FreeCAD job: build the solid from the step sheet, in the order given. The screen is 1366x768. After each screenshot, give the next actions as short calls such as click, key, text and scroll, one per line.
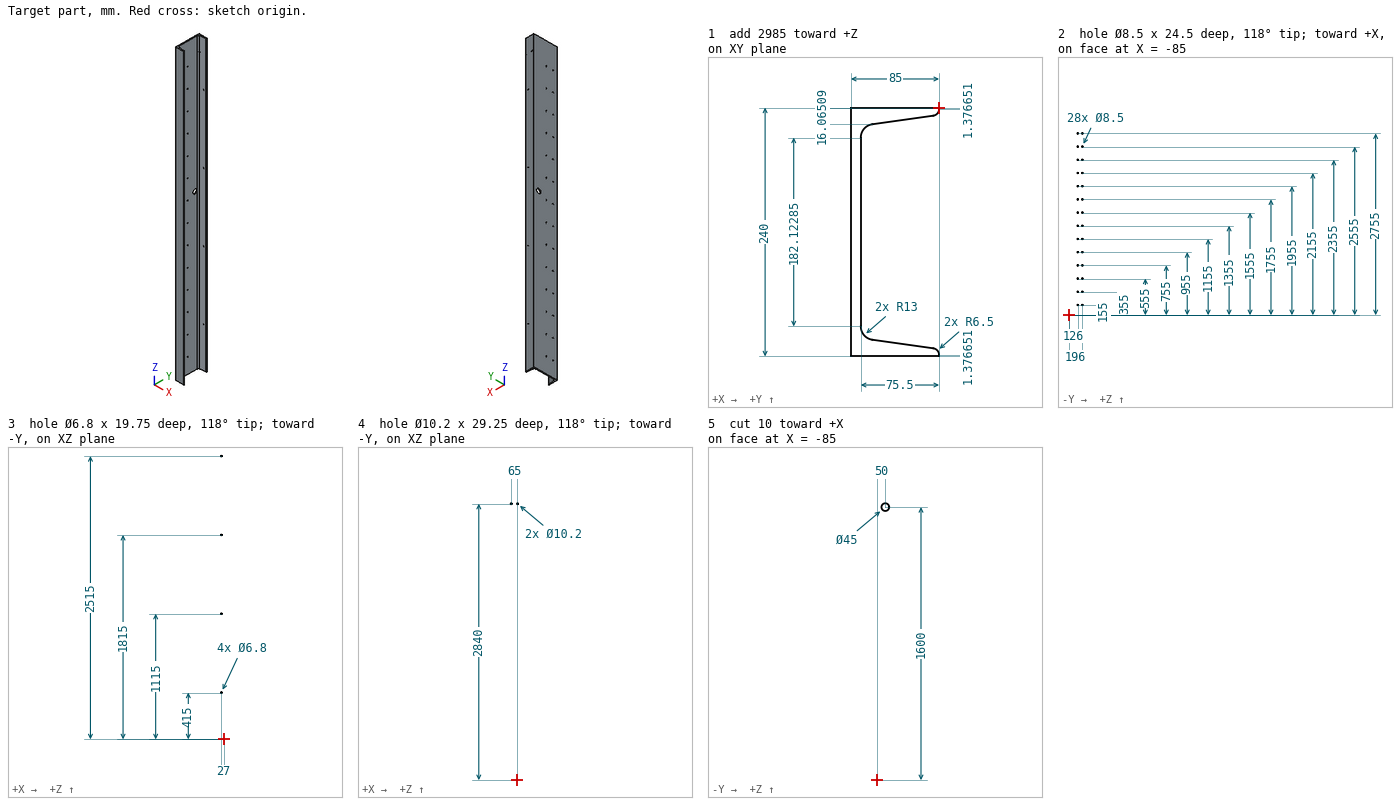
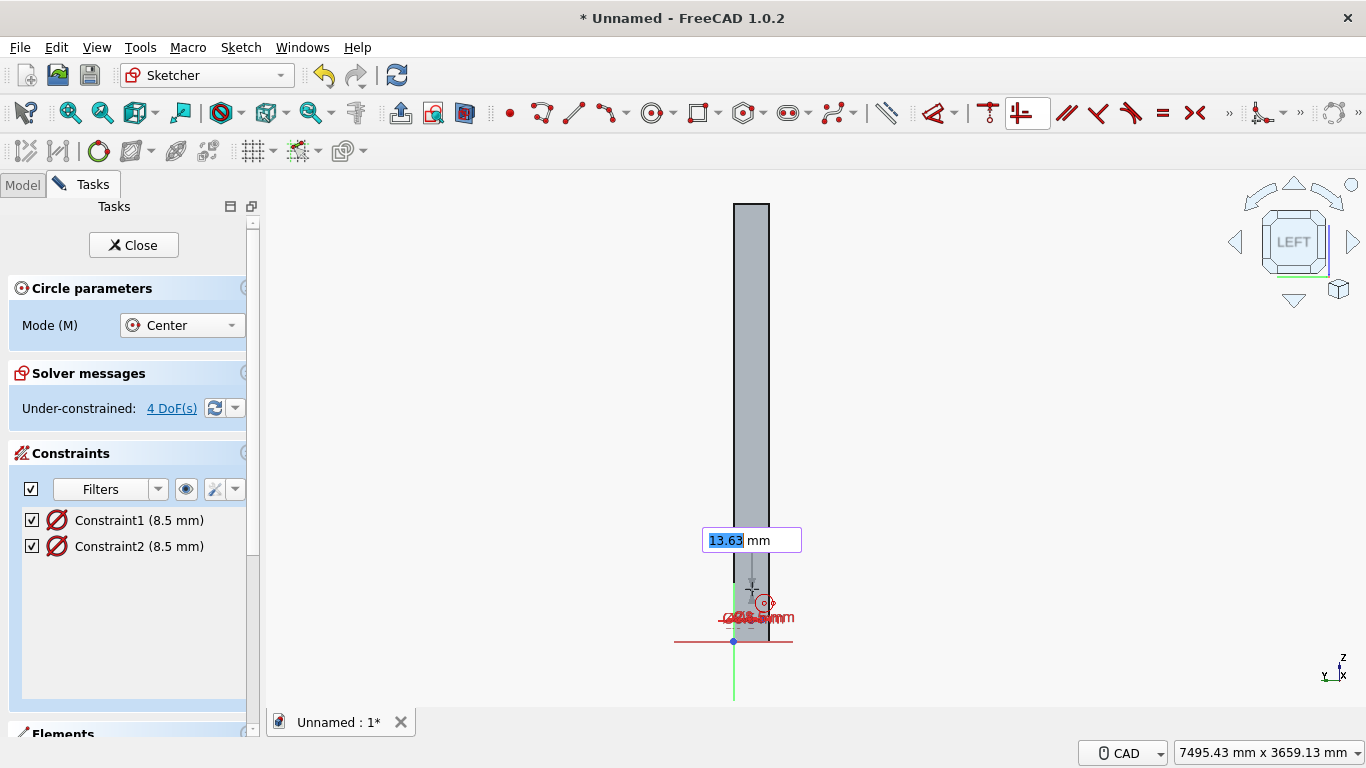
text(8.5)
key(Return)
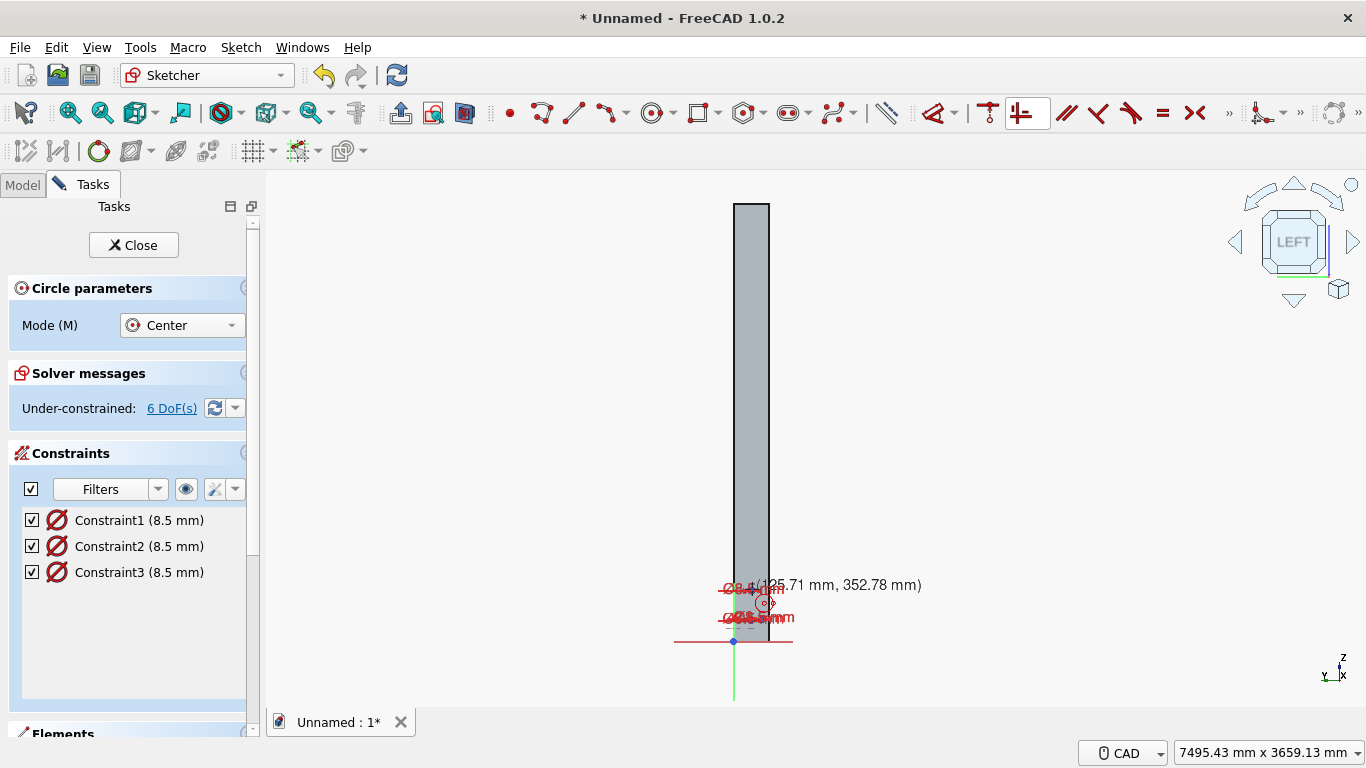
scroll(762, 590, up, 18)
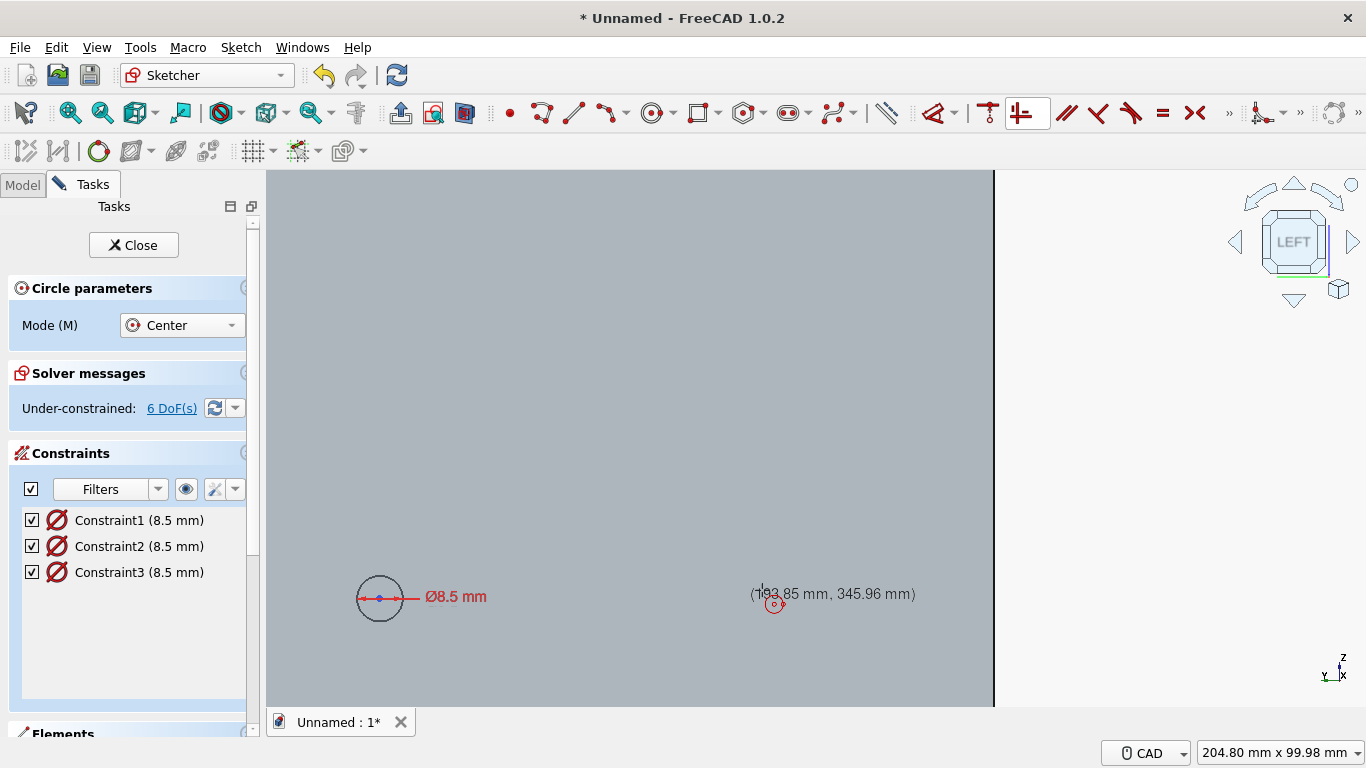
scroll(762, 590, down, 18)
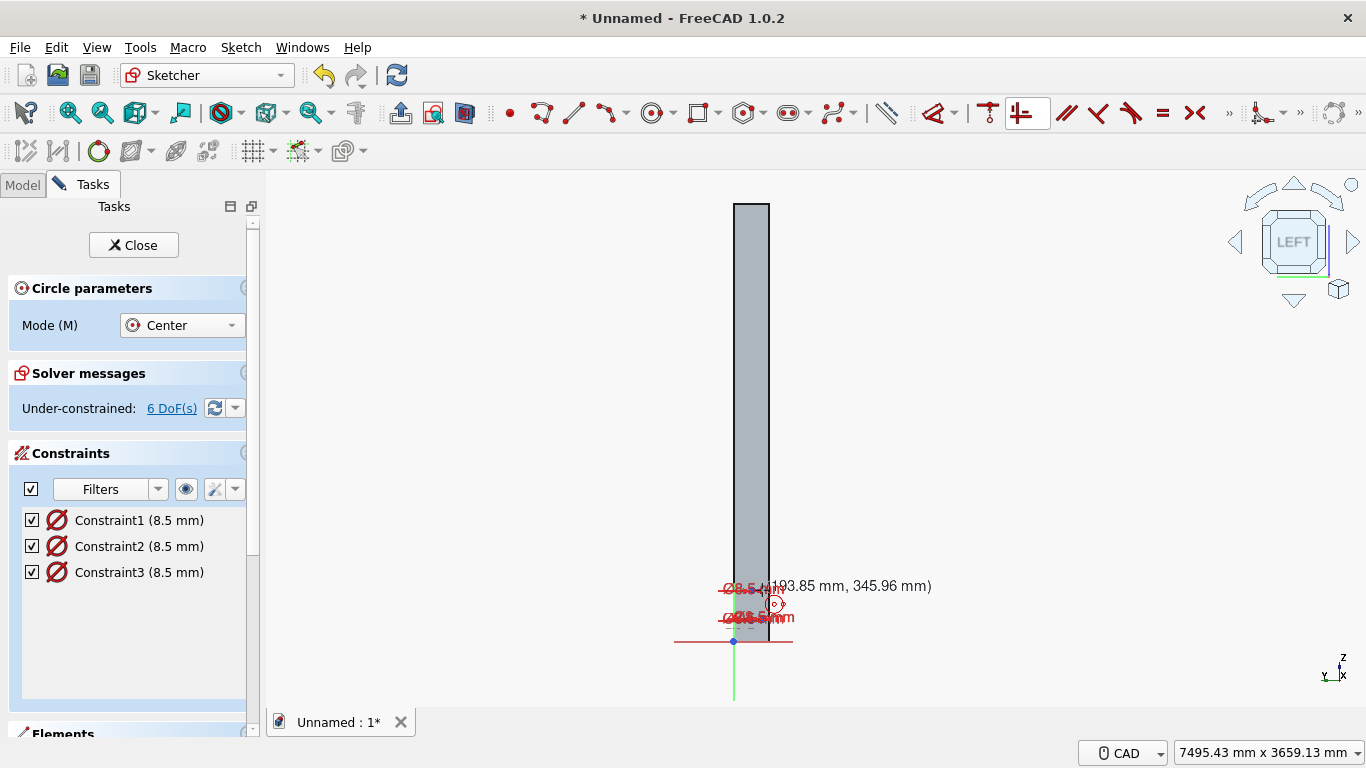
scroll(762, 590, up, 3)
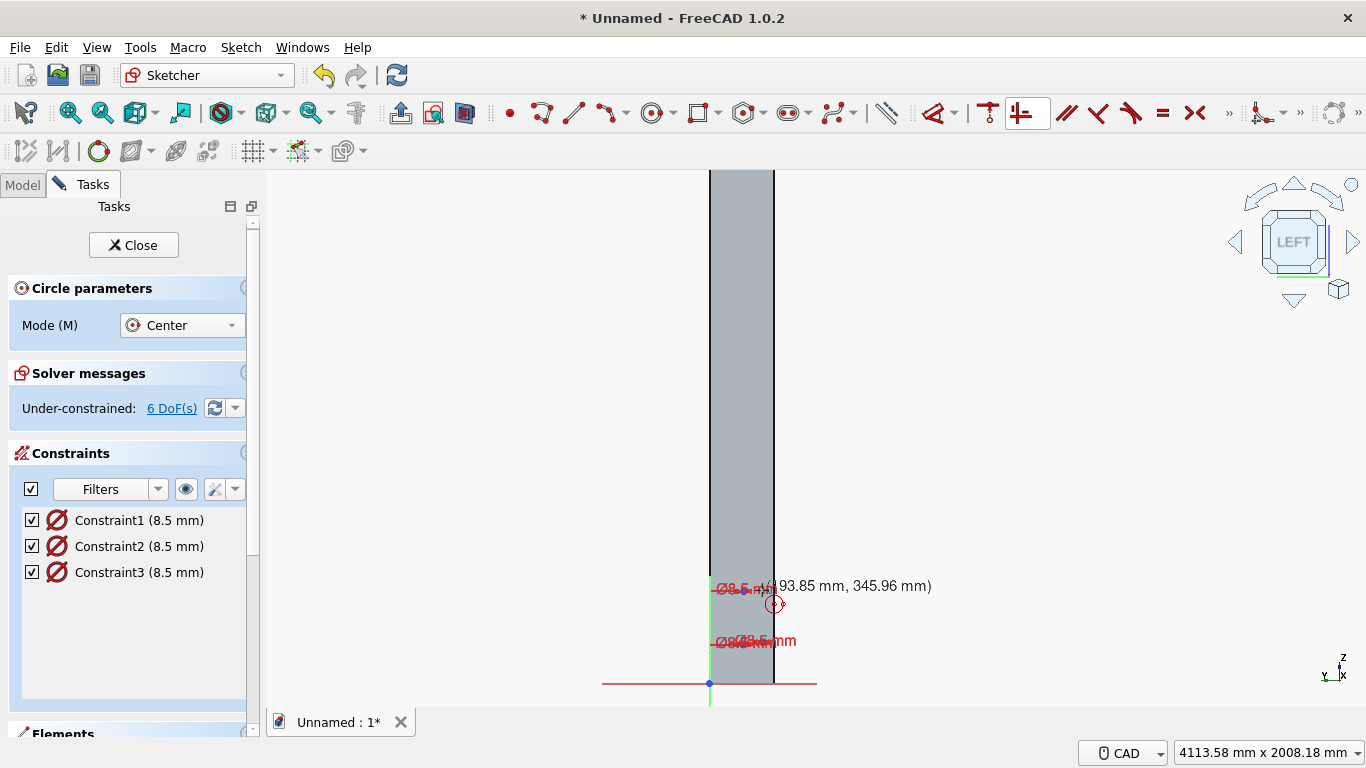
click(762, 589)
move(763, 588)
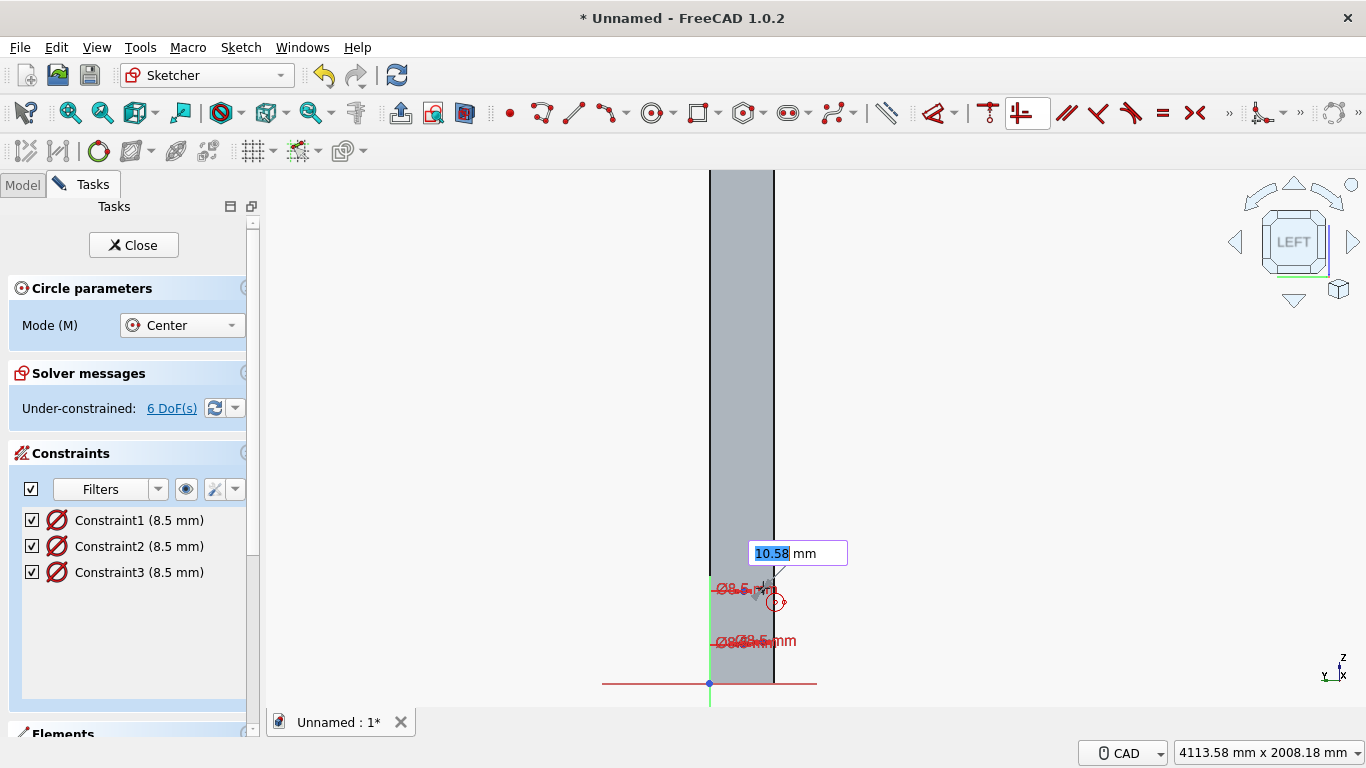
text(8.5)
key(Return)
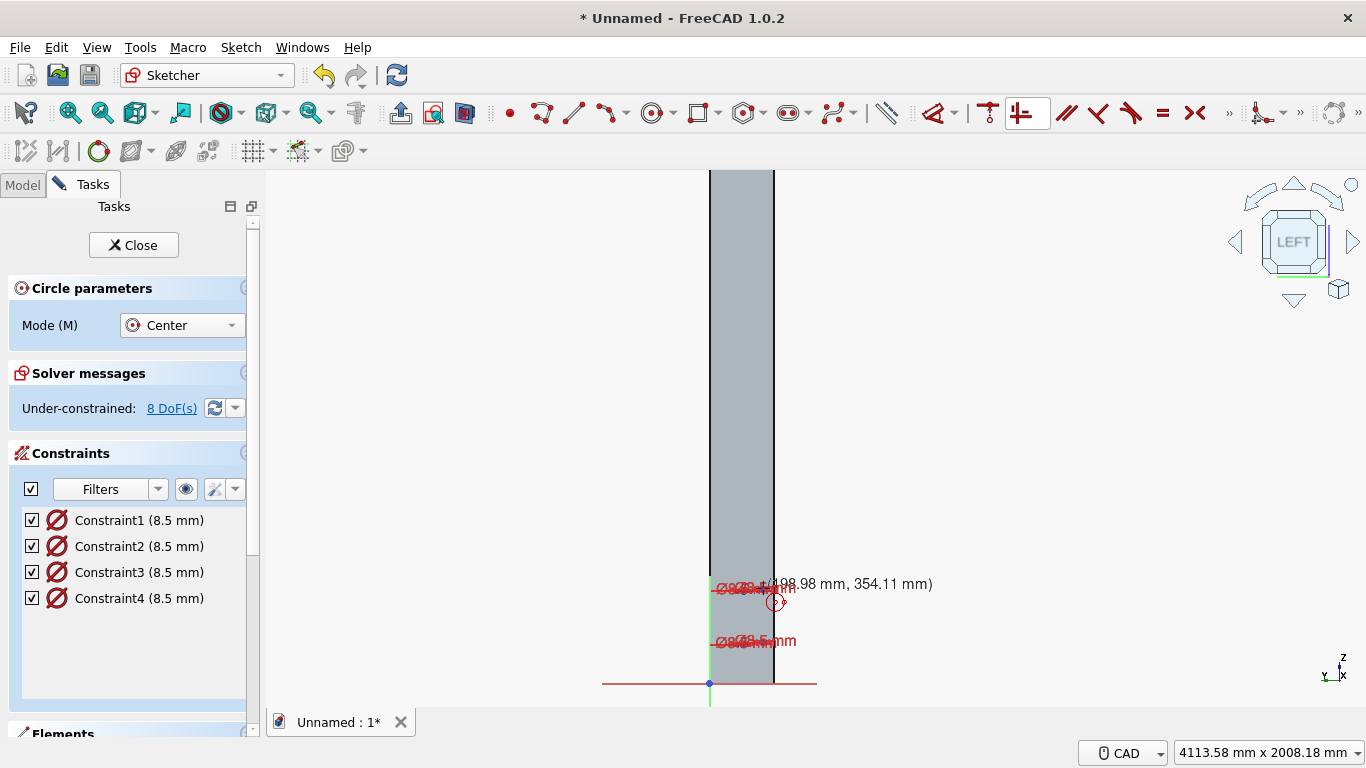
scroll(743, 535, up, 15)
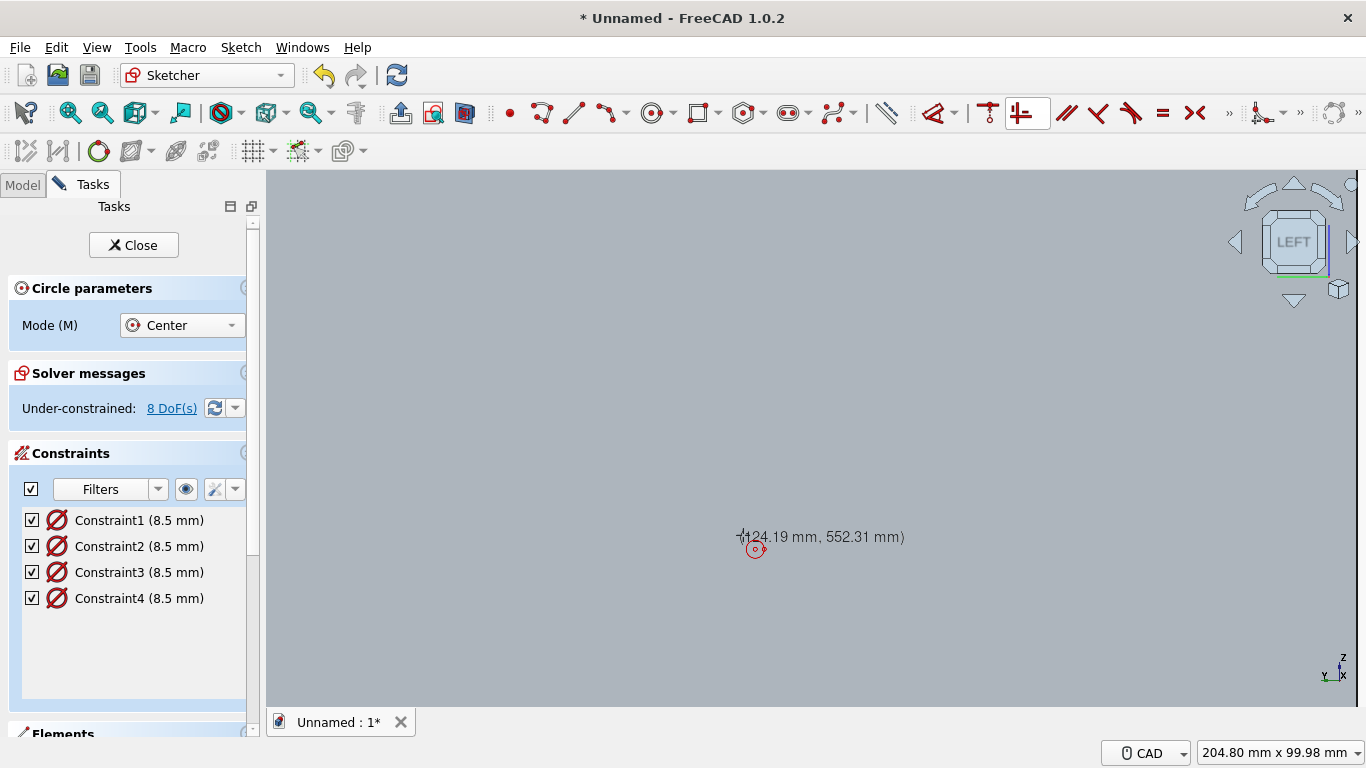
scroll(751, 560, down, 18)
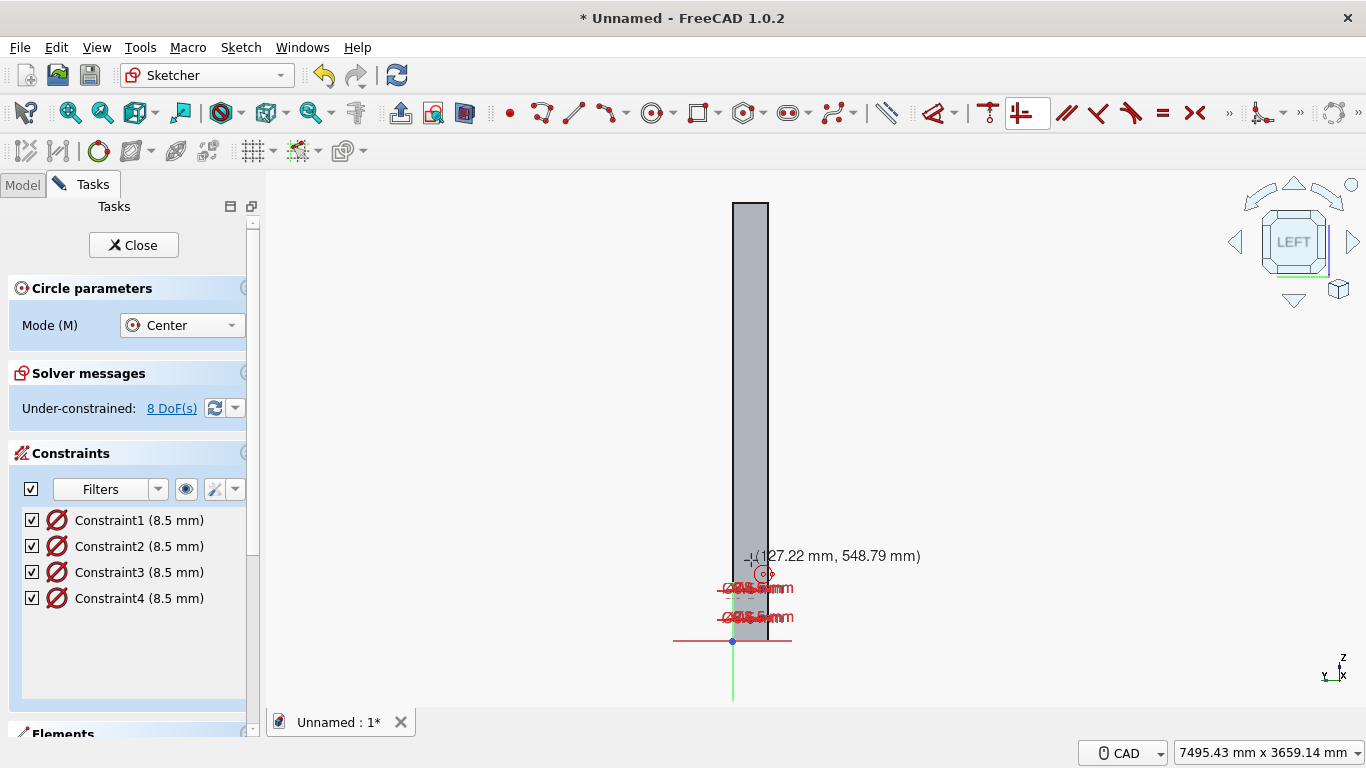
click(751, 560)
move(752, 559)